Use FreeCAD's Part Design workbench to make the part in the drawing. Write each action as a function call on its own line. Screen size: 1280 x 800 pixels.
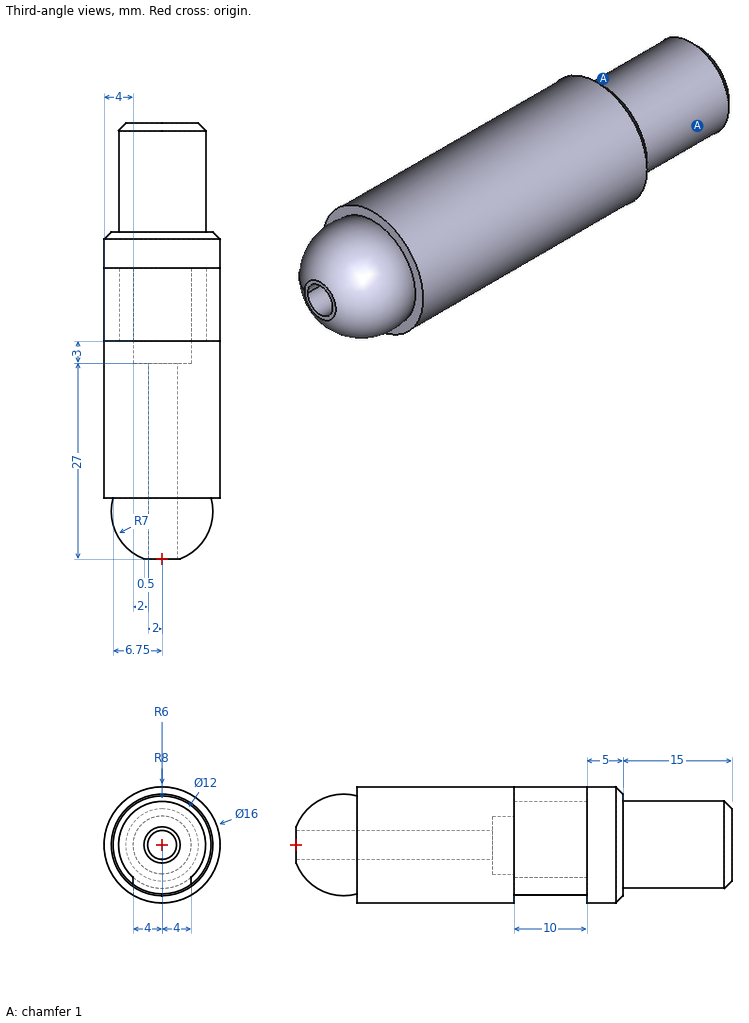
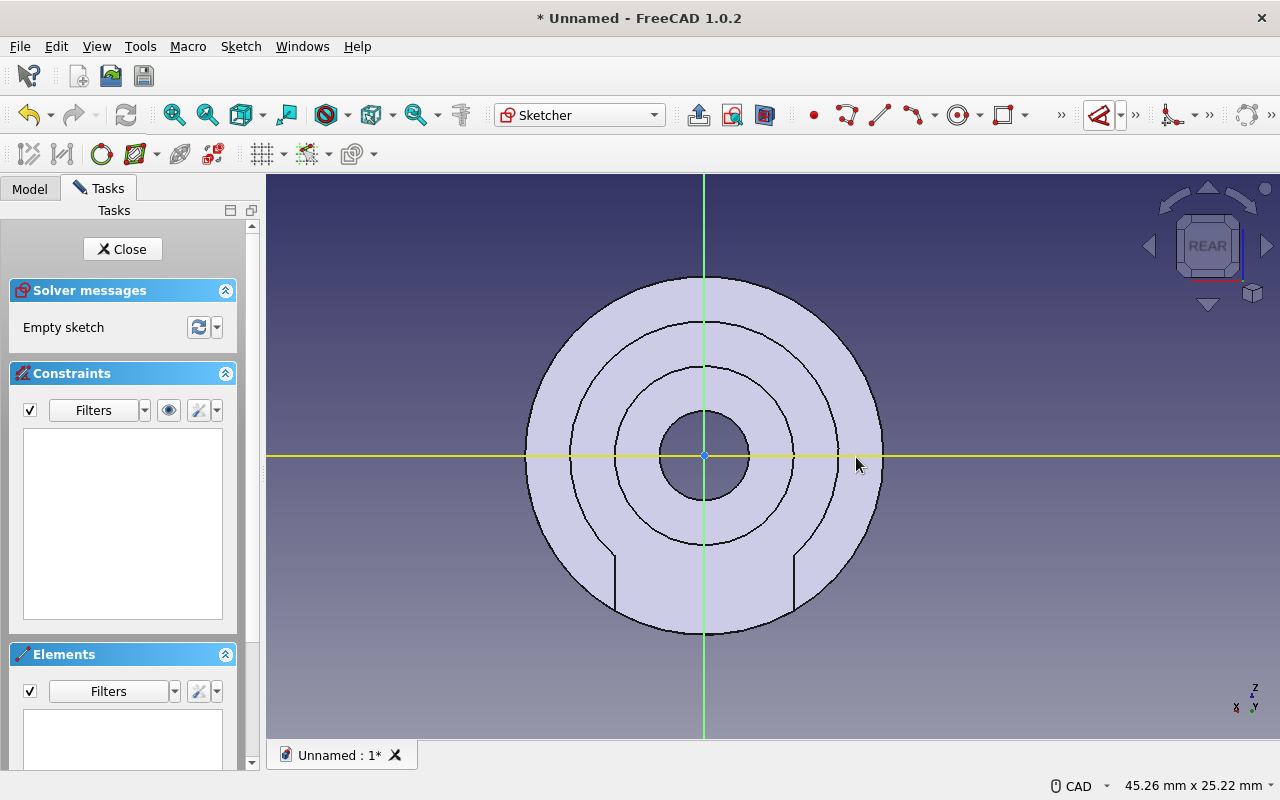
click(958, 116)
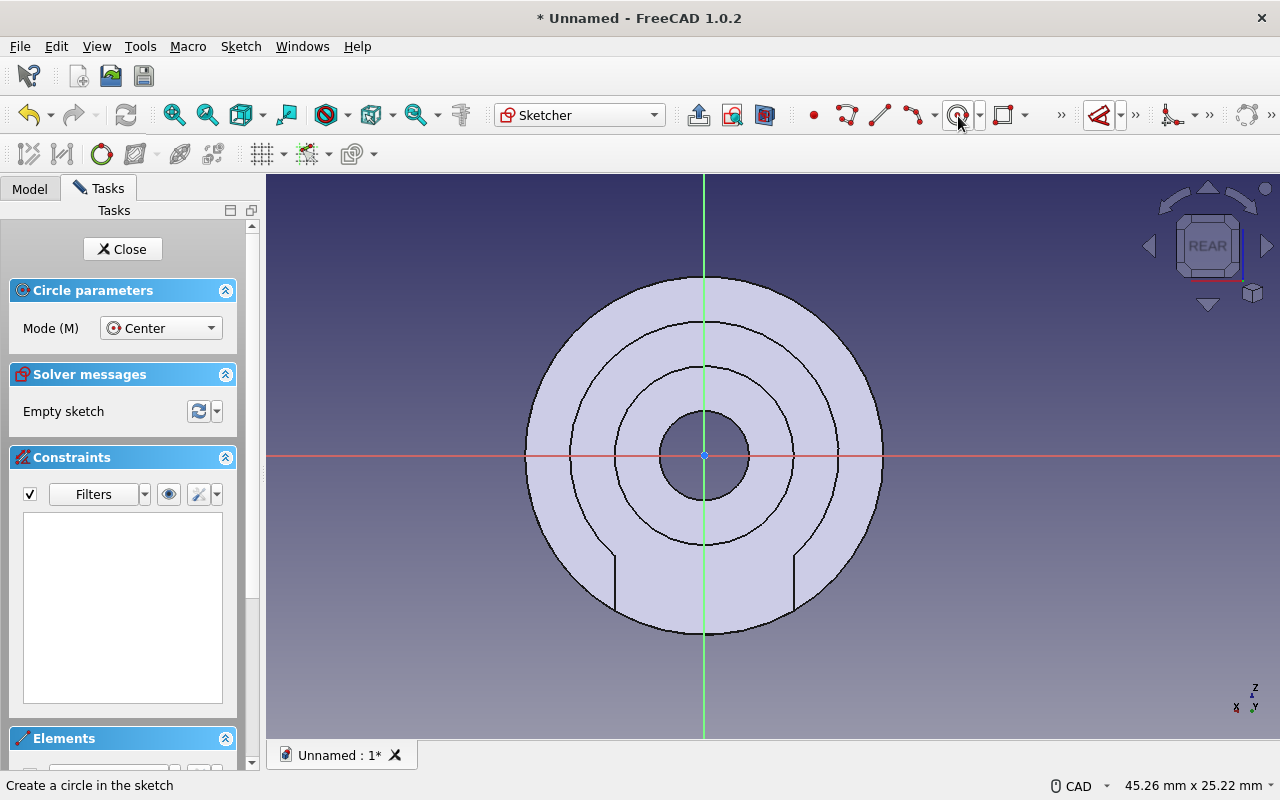
click(704, 456)
click(831, 329)
key(Escape)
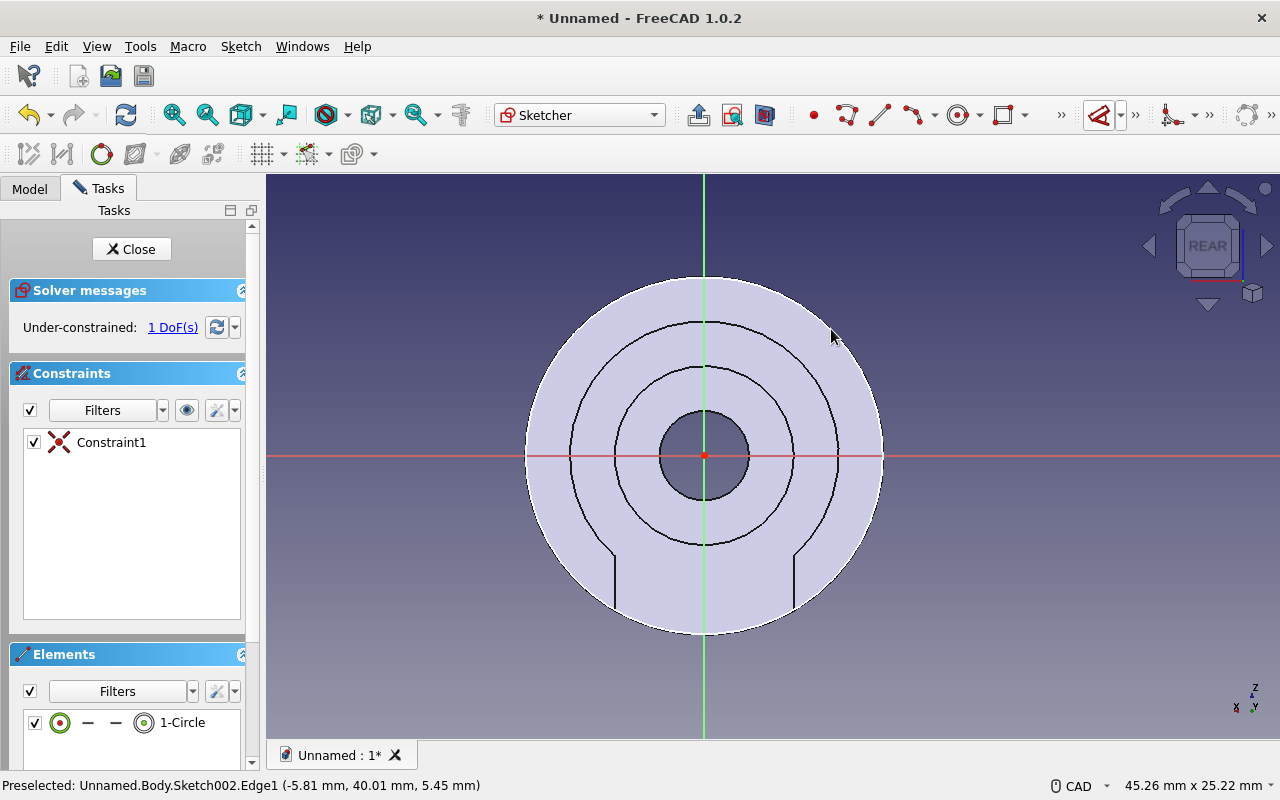
click(830, 329)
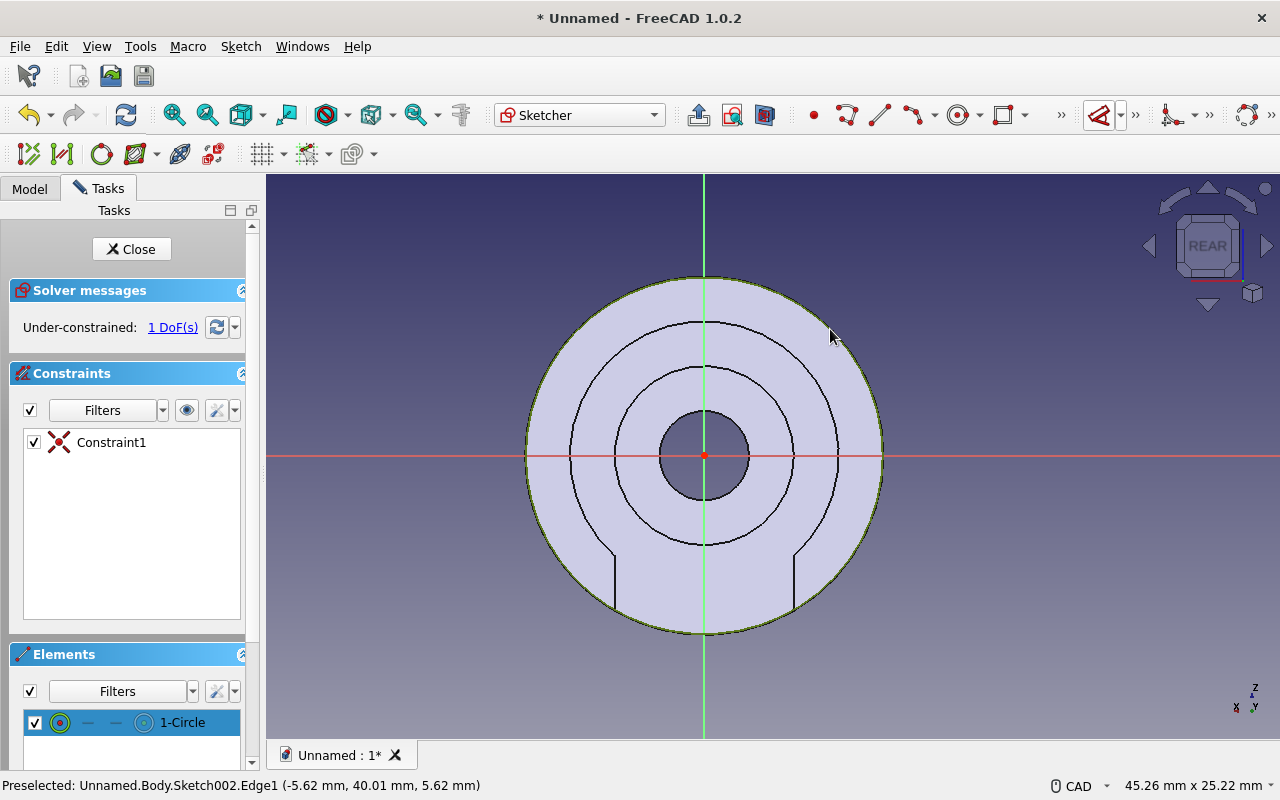
click(1120, 116)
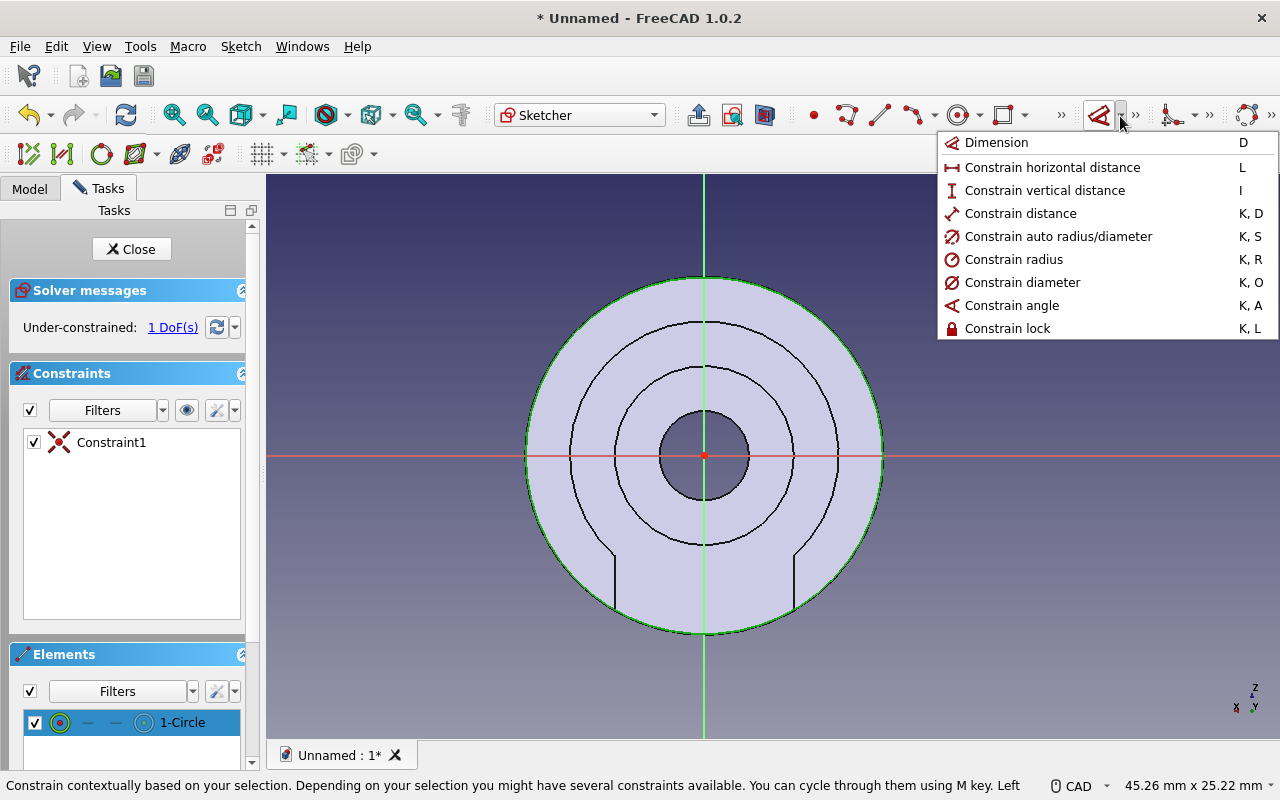
click(1108, 282)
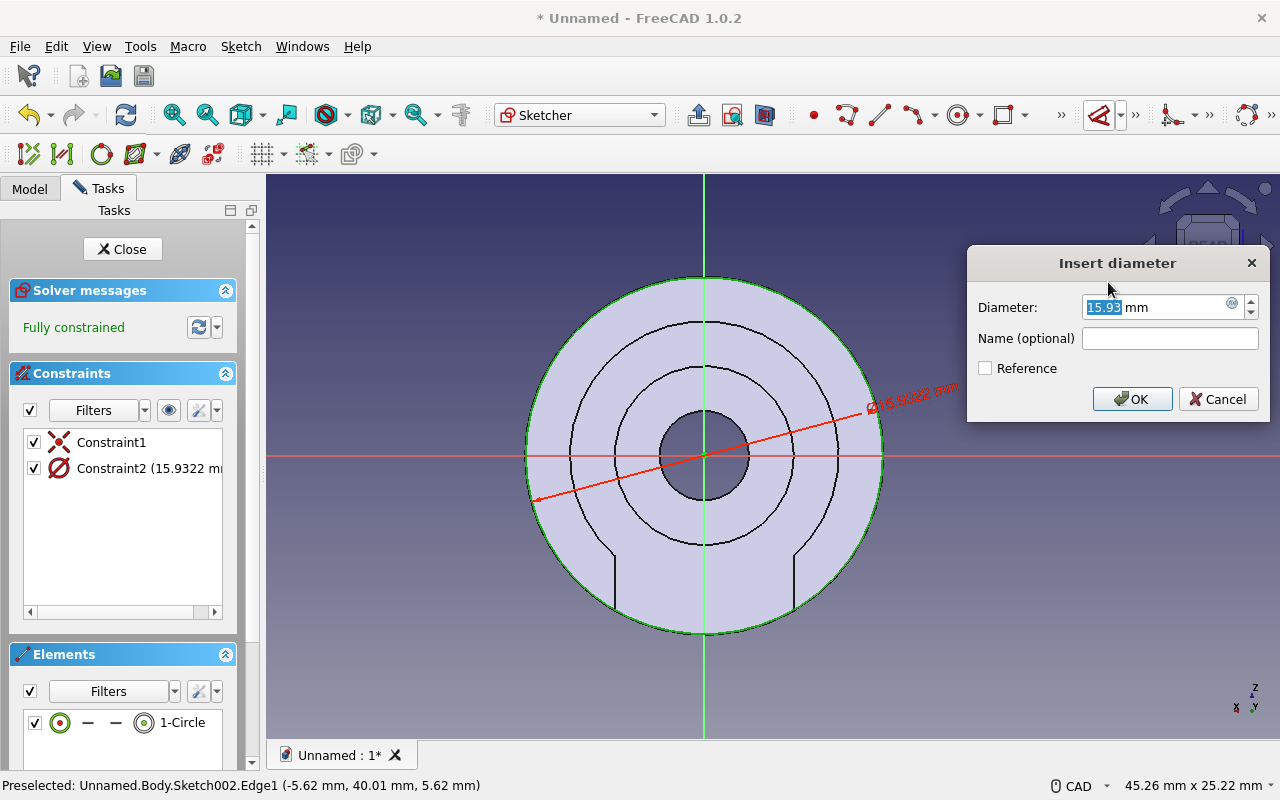
text(16)
key(Return)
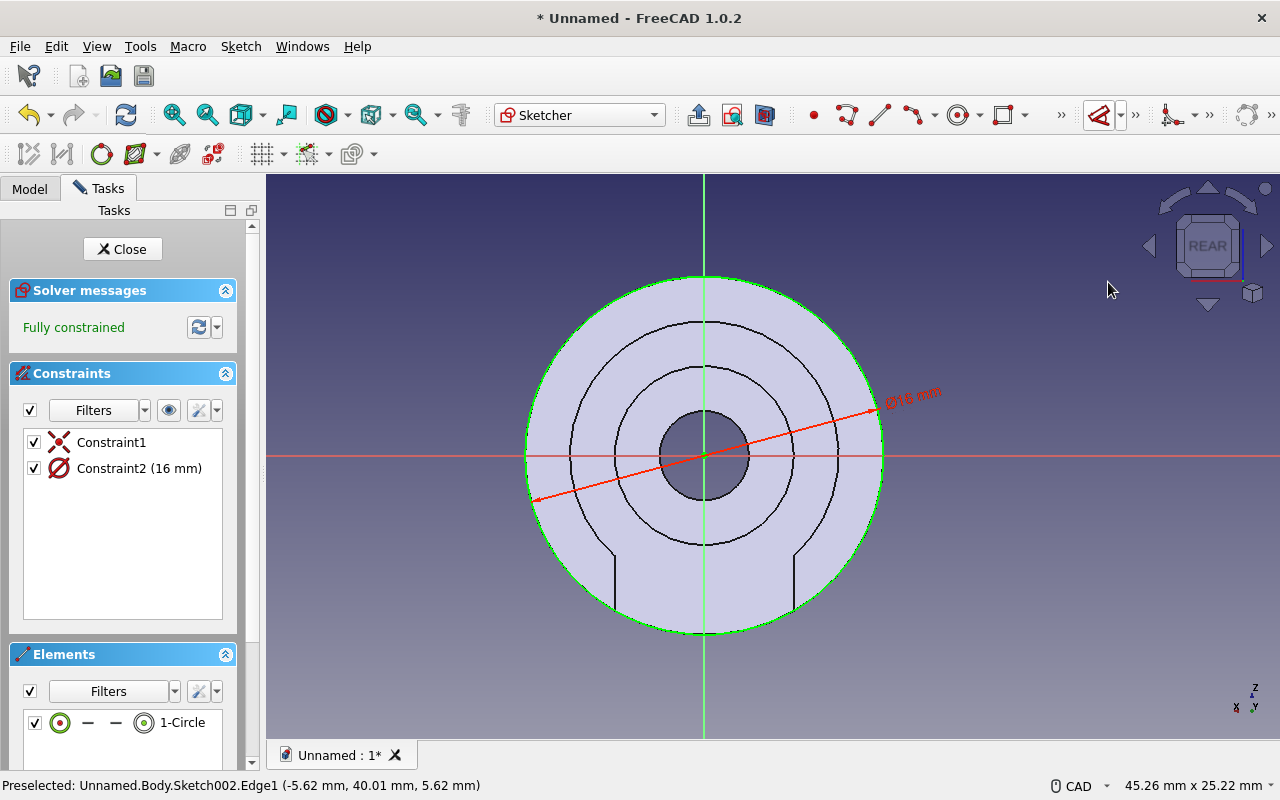
click(123, 249)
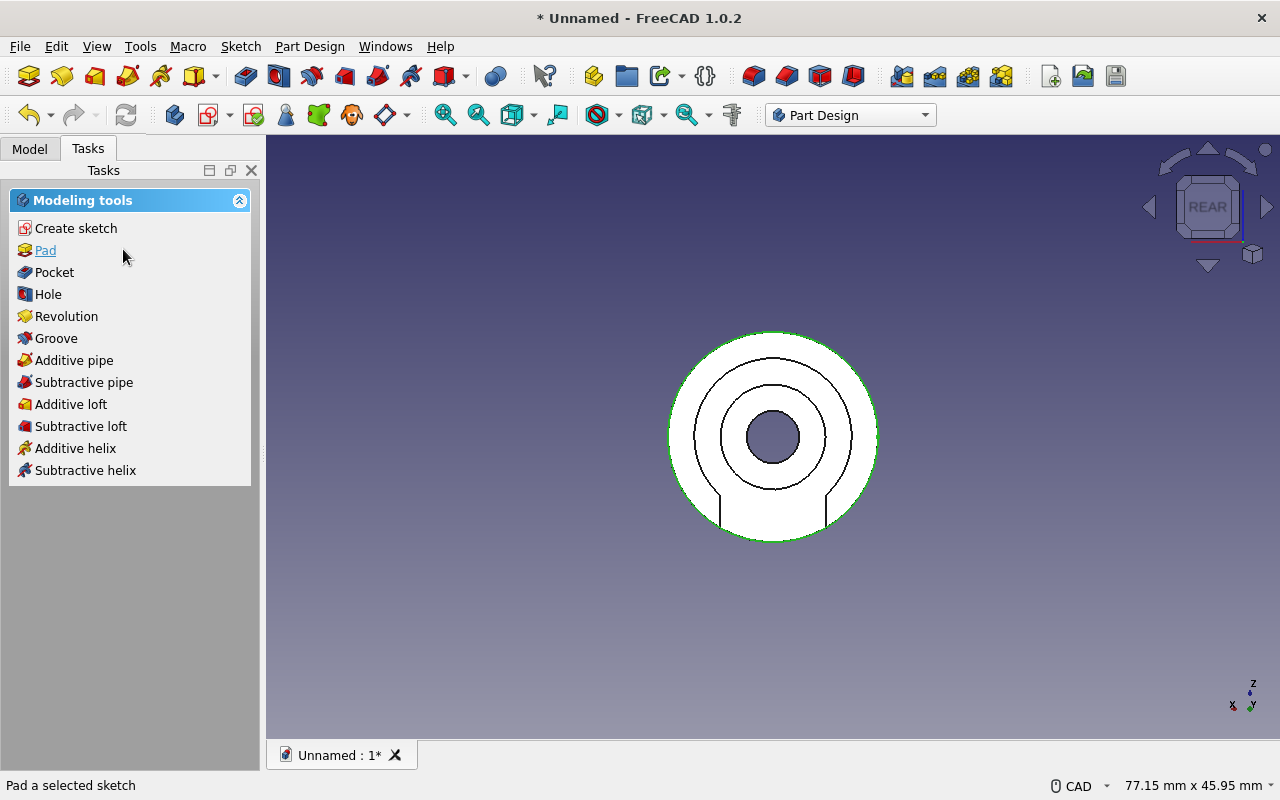
click(29, 76)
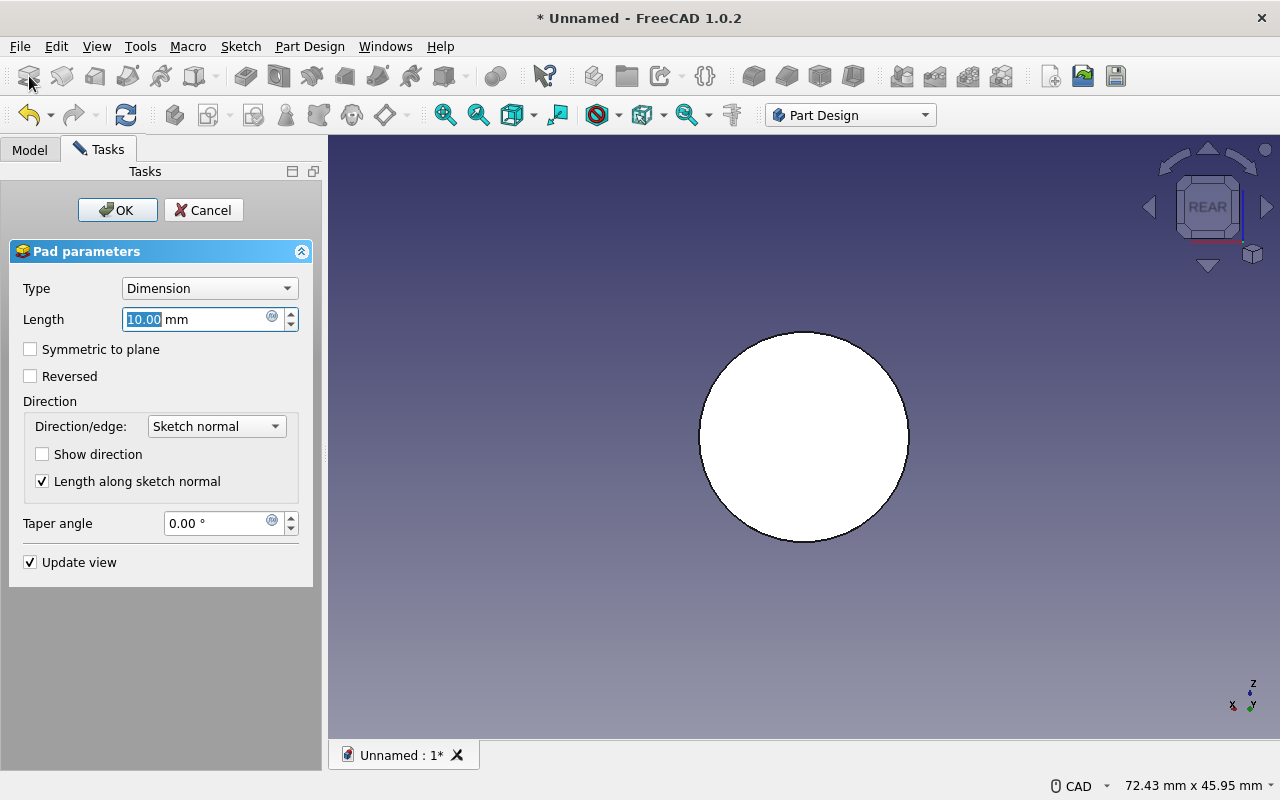
text(5)
key(Tab)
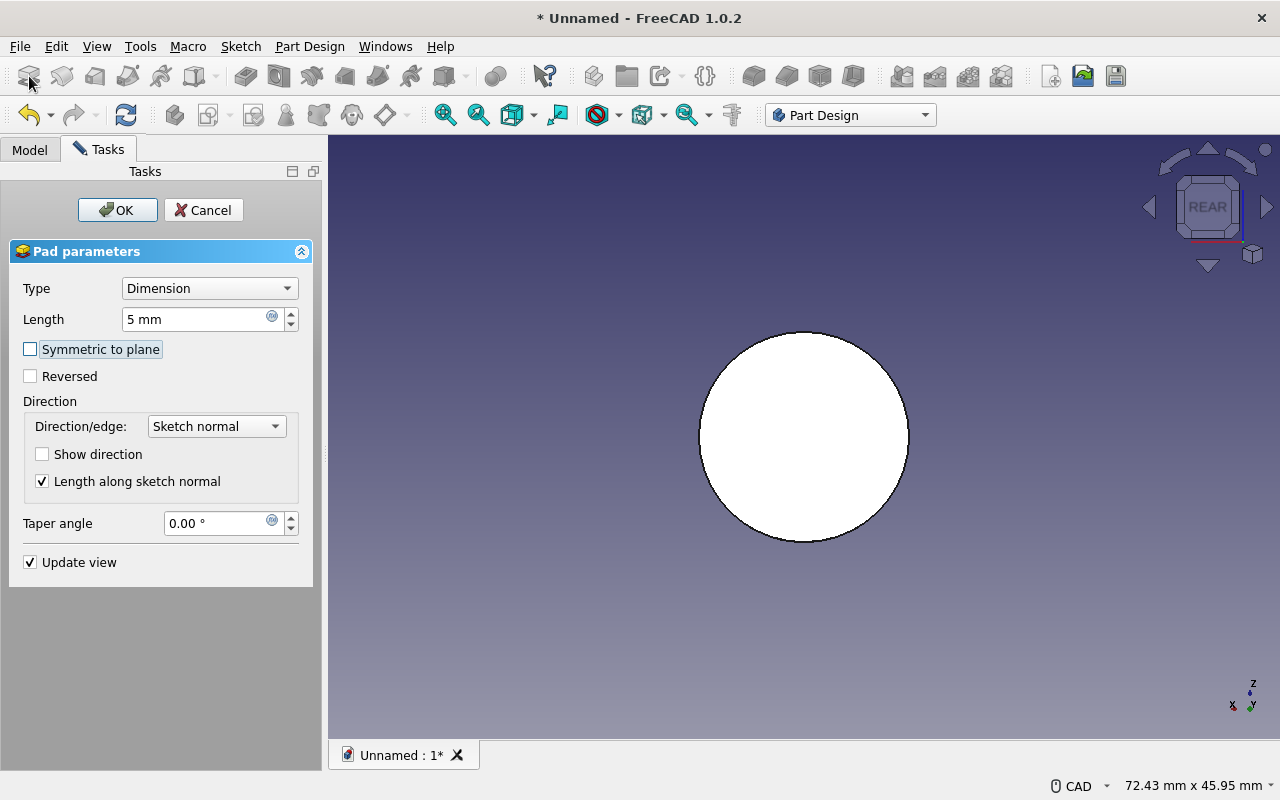
click(118, 210)